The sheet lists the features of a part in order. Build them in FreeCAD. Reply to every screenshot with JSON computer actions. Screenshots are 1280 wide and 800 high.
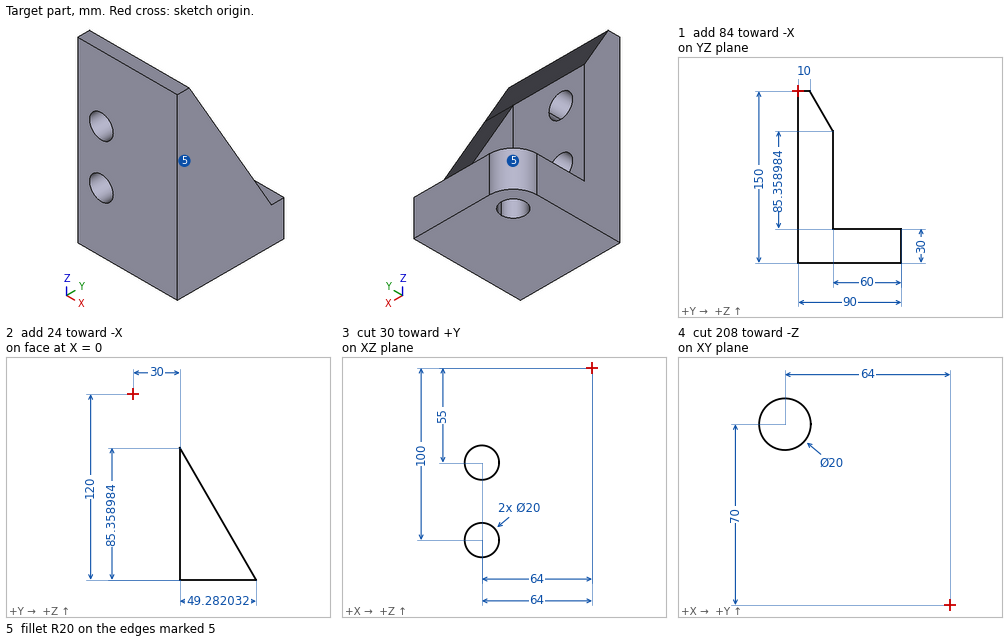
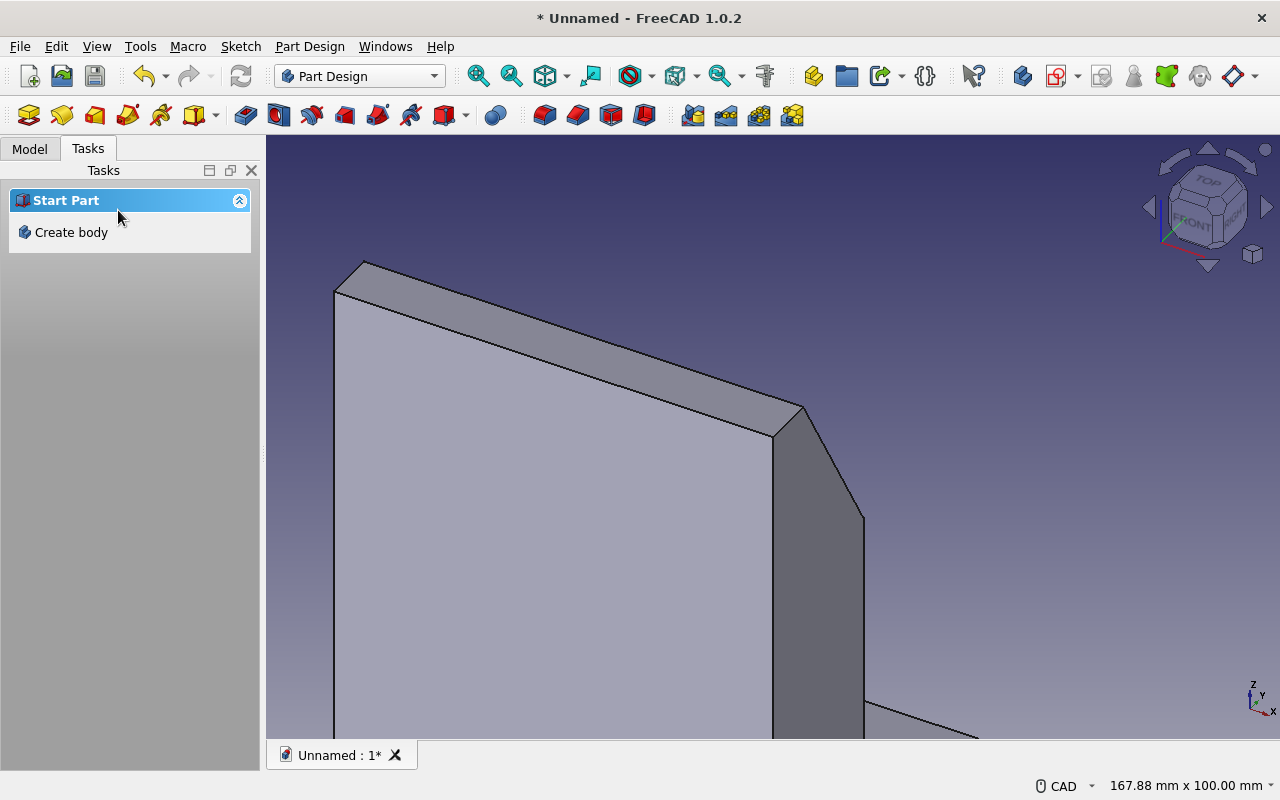
{"action": "left_click", "coordinate": [479, 76]}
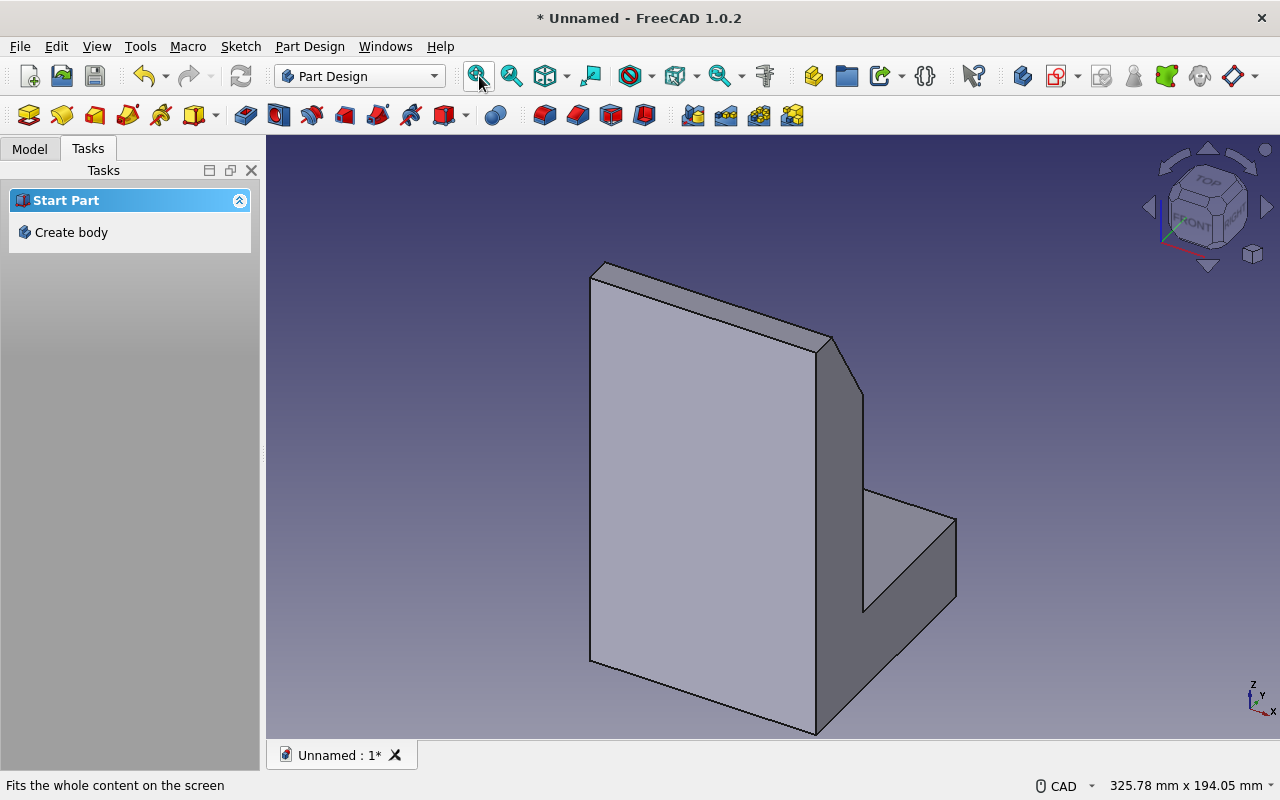
{"action": "left_click", "coordinate": [926, 598]}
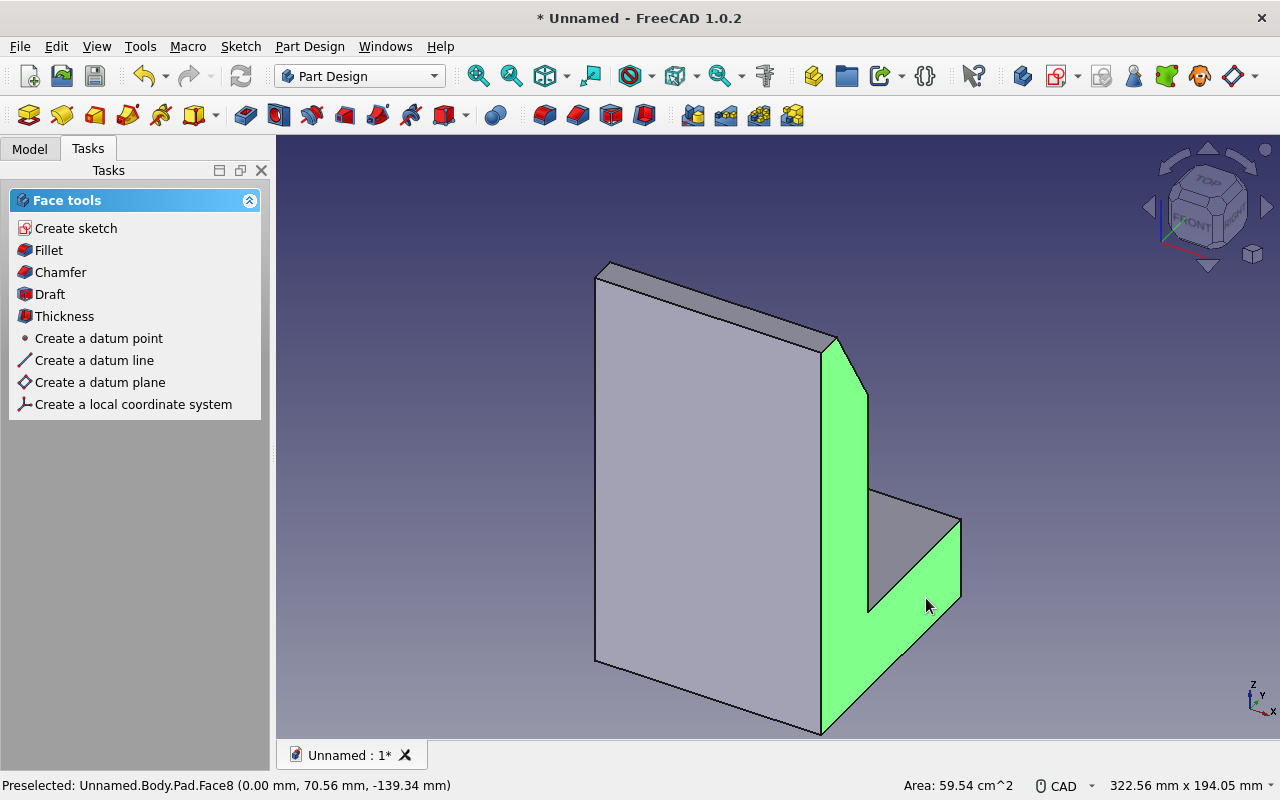
{"action": "left_click", "coordinate": [1056, 76]}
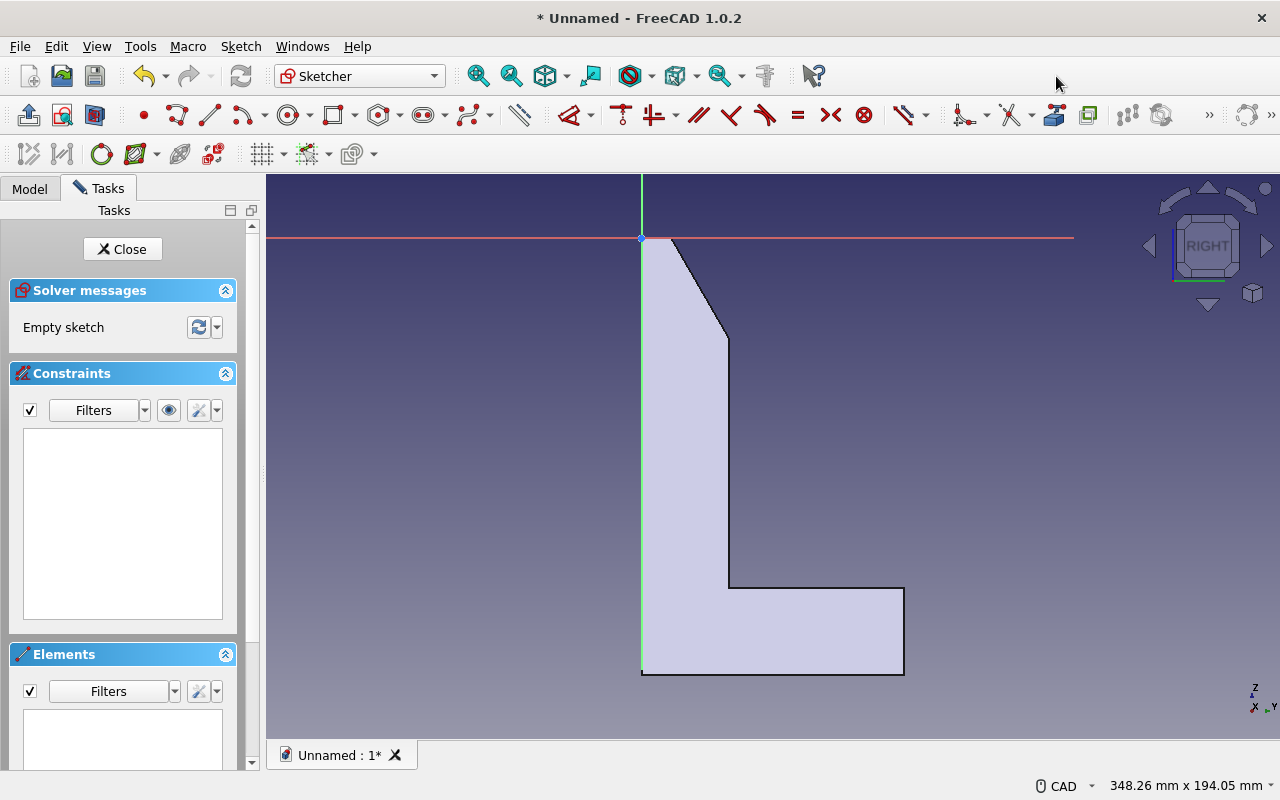
{"action": "left_click", "coordinate": [177, 116]}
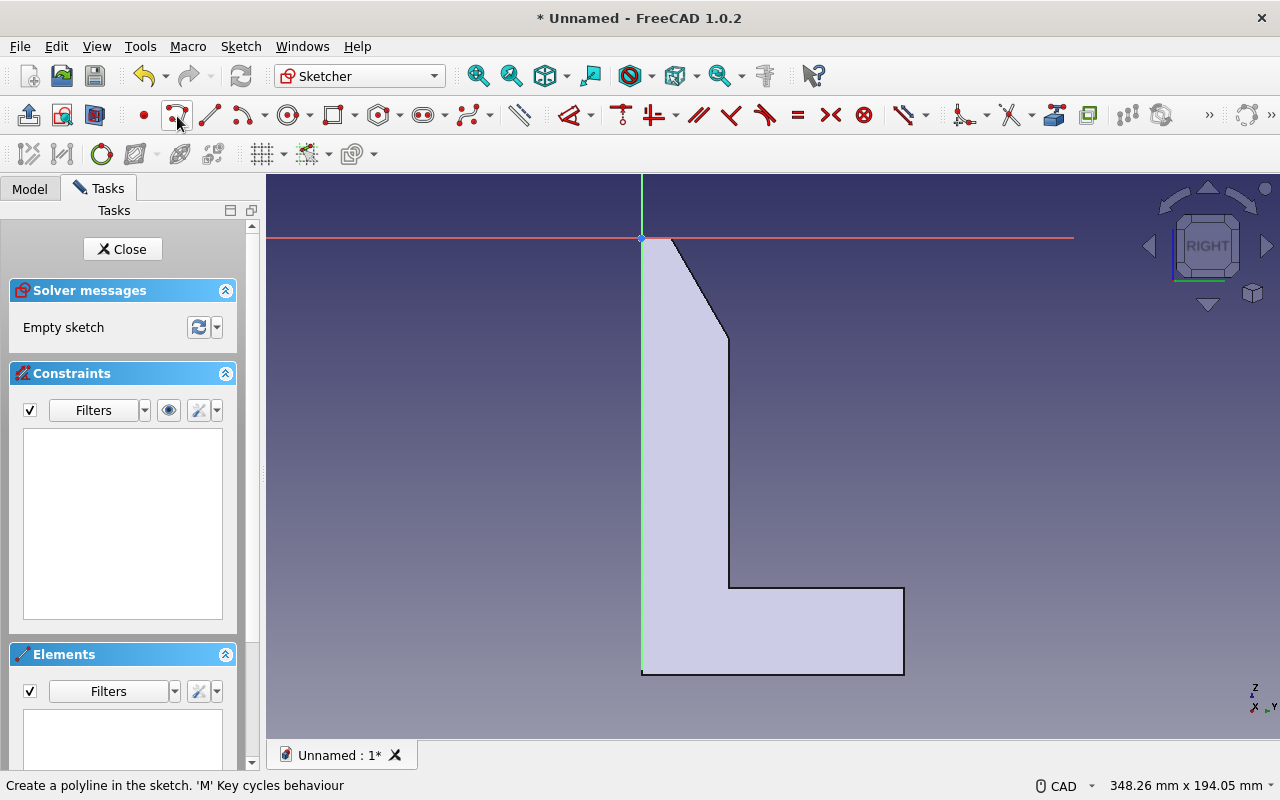
{"action": "left_click", "coordinate": [729, 339]}
{"action": "left_click", "coordinate": [729, 588]}
{"action": "left_click", "coordinate": [873, 588]}
{"action": "left_click", "coordinate": [729, 340]}
{"action": "key", "text": "Escape"}
{"action": "key", "text": "Escape"}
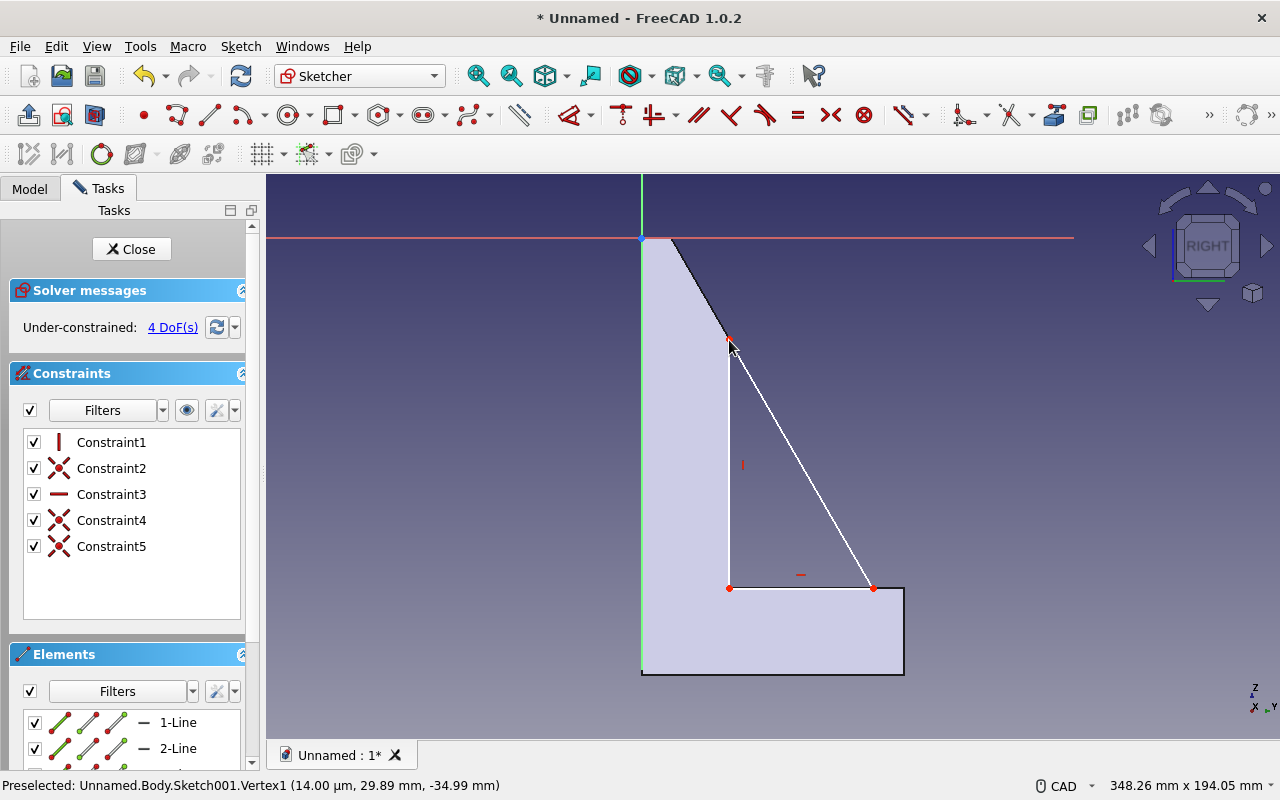
{"action": "left_click", "coordinate": [568, 116]}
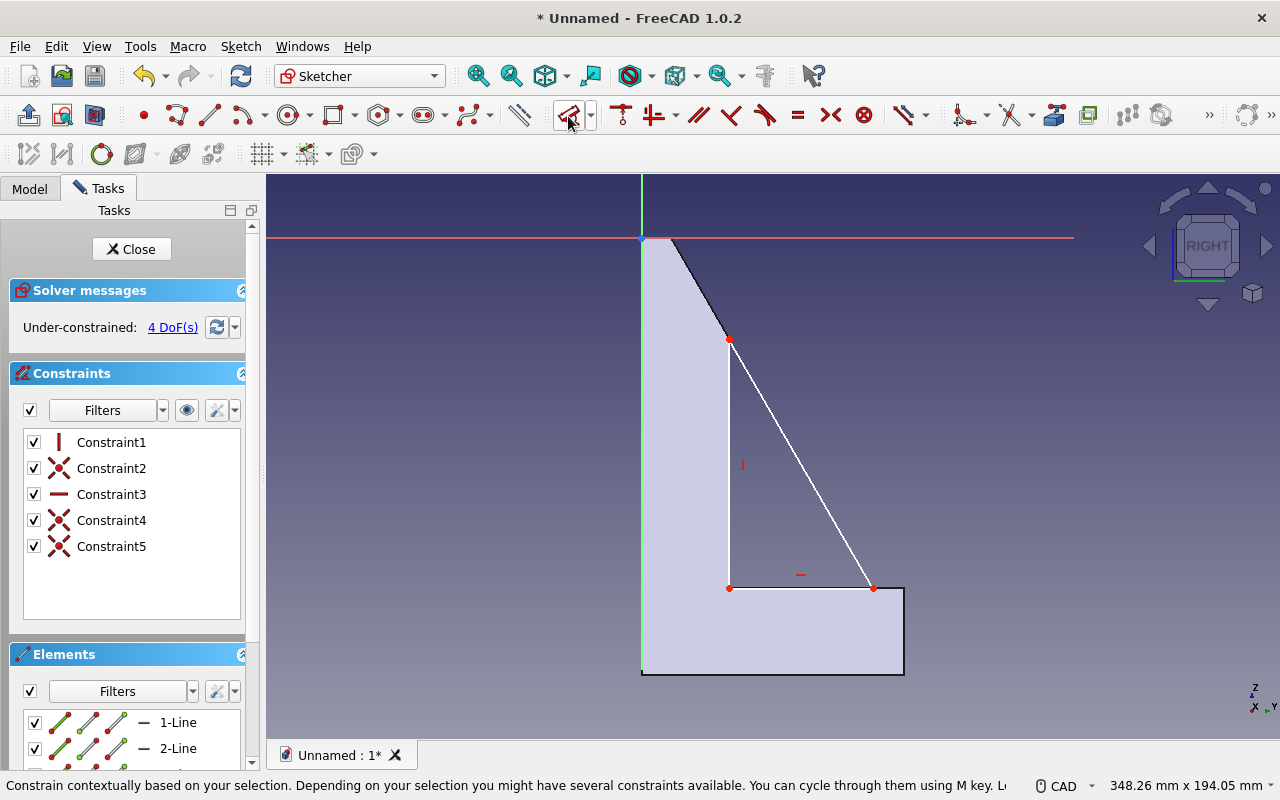
{"action": "left_click", "coordinate": [729, 340]}
{"action": "left_click", "coordinate": [685, 204]}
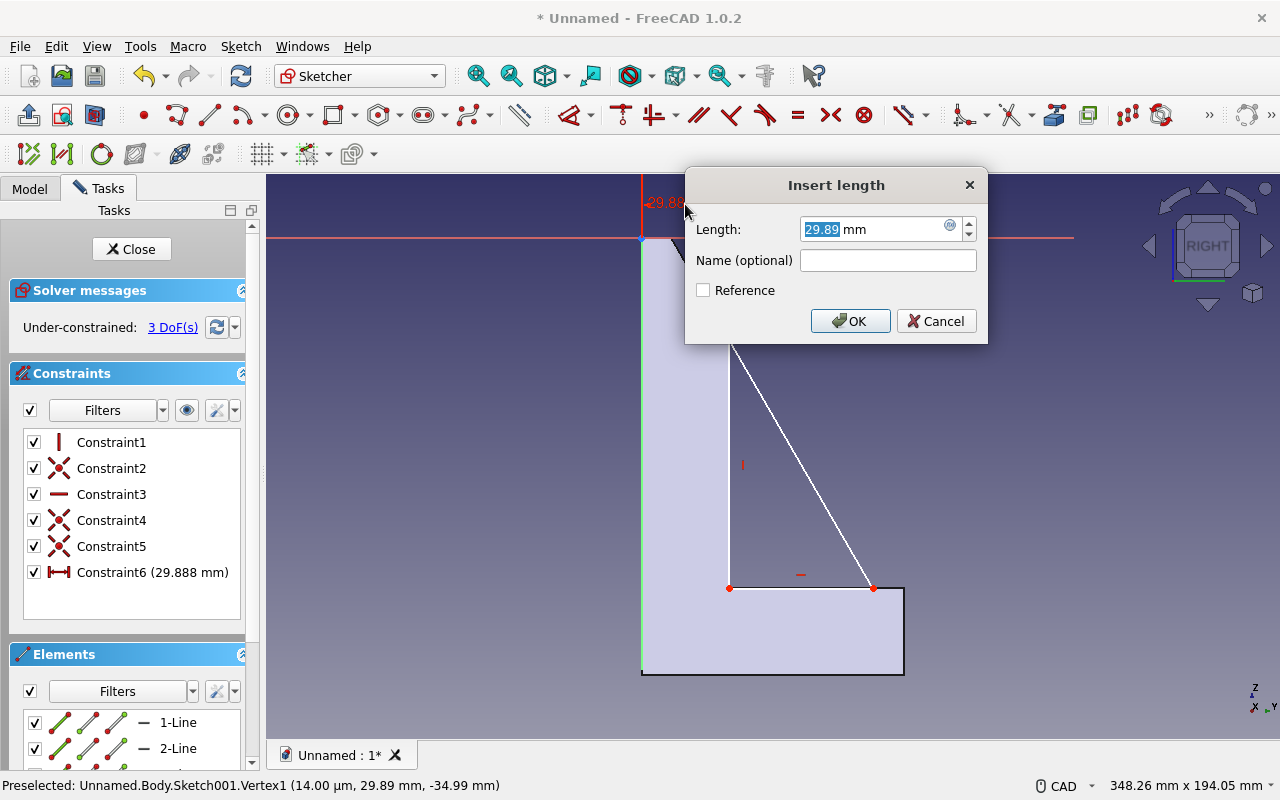
{"action": "type", "text": "30"}
{"action": "key", "text": "Return"}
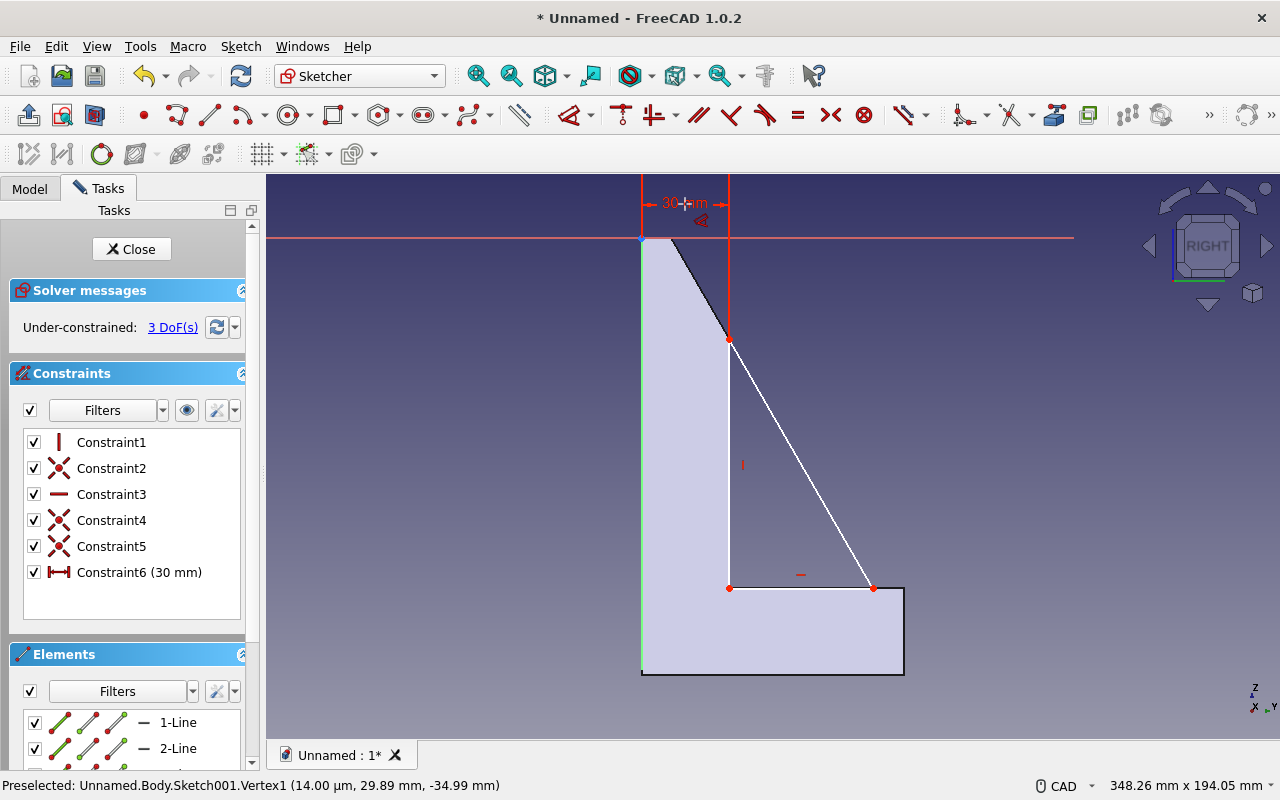
{"action": "left_click", "coordinate": [729, 589]}
{"action": "left_click", "coordinate": [608, 414]}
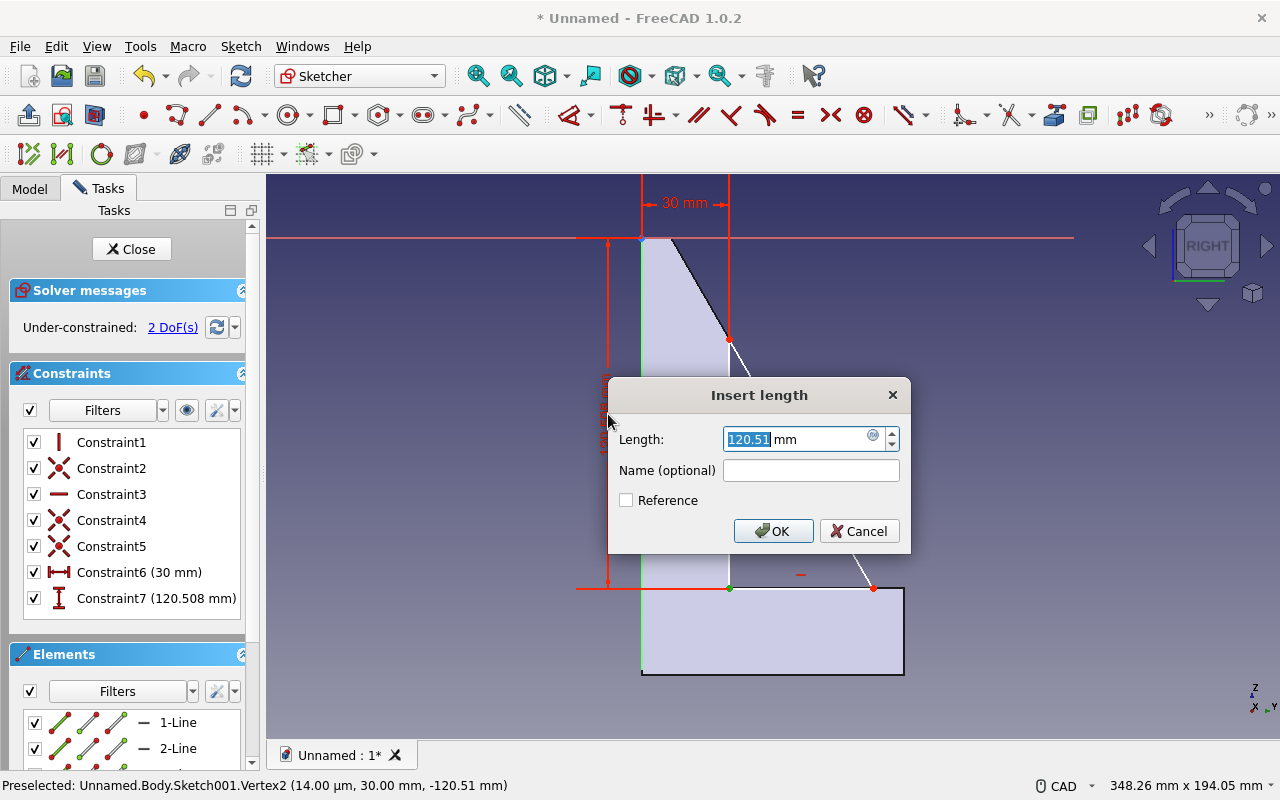
{"action": "type", "text": "120"}
{"action": "key", "text": "Return"}